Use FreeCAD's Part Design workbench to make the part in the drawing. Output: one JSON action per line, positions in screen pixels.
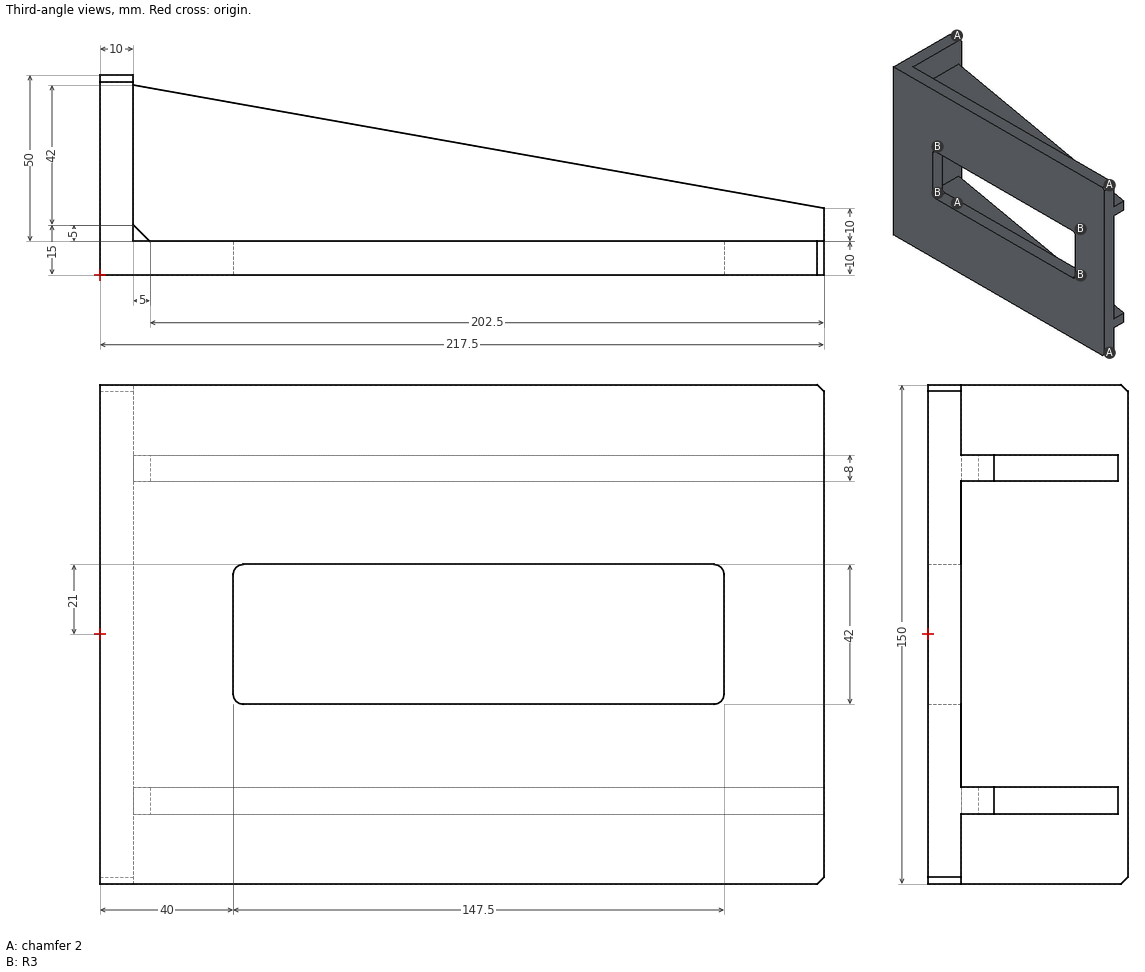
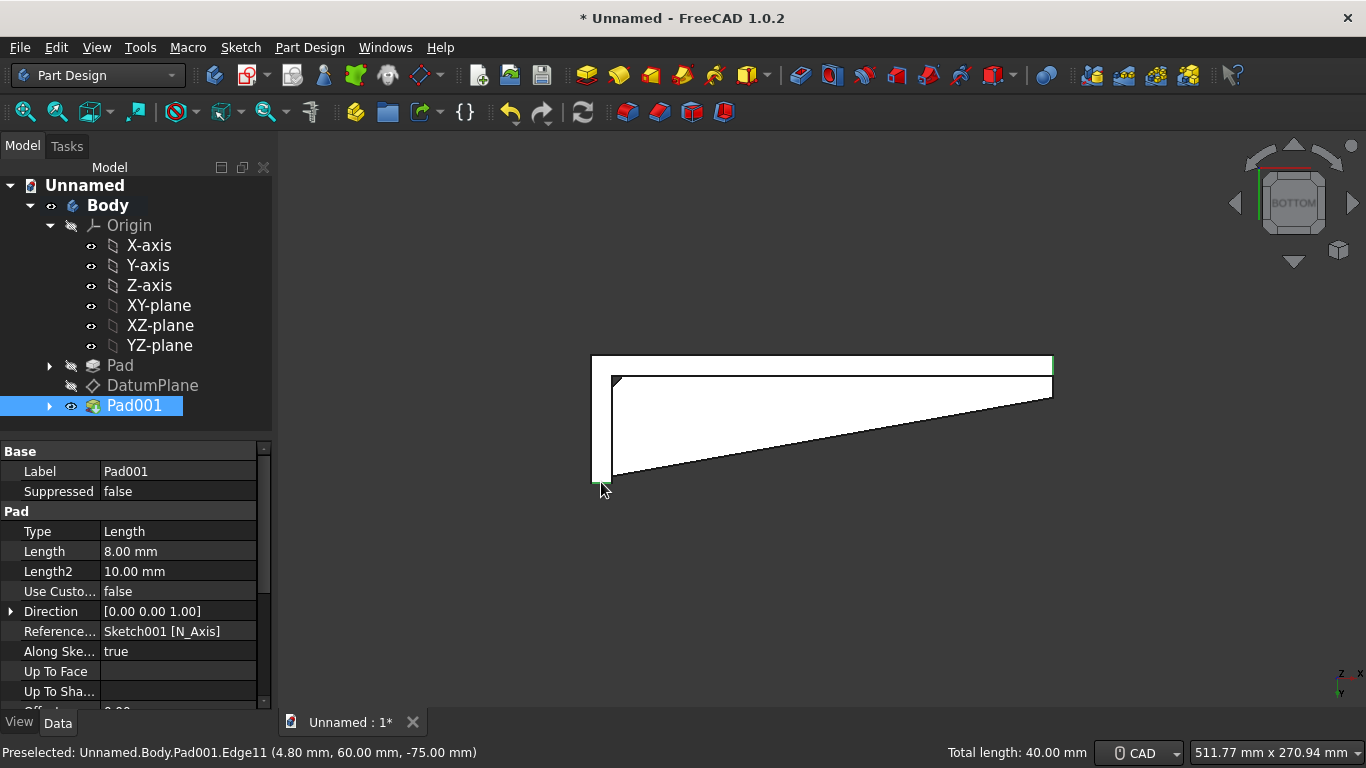
{"action": "left_click", "coordinate": [660, 112]}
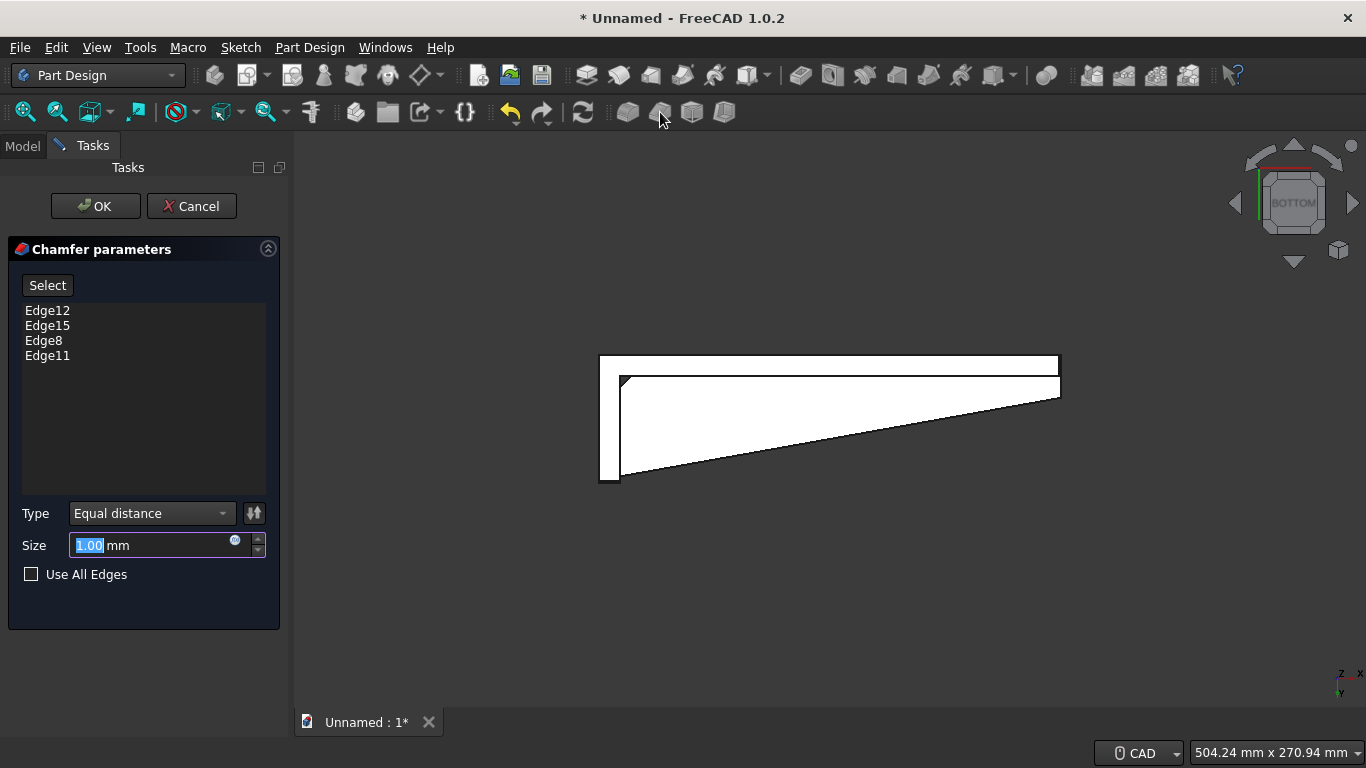
{"action": "type", "text": "2"}
{"action": "key", "text": "Tab"}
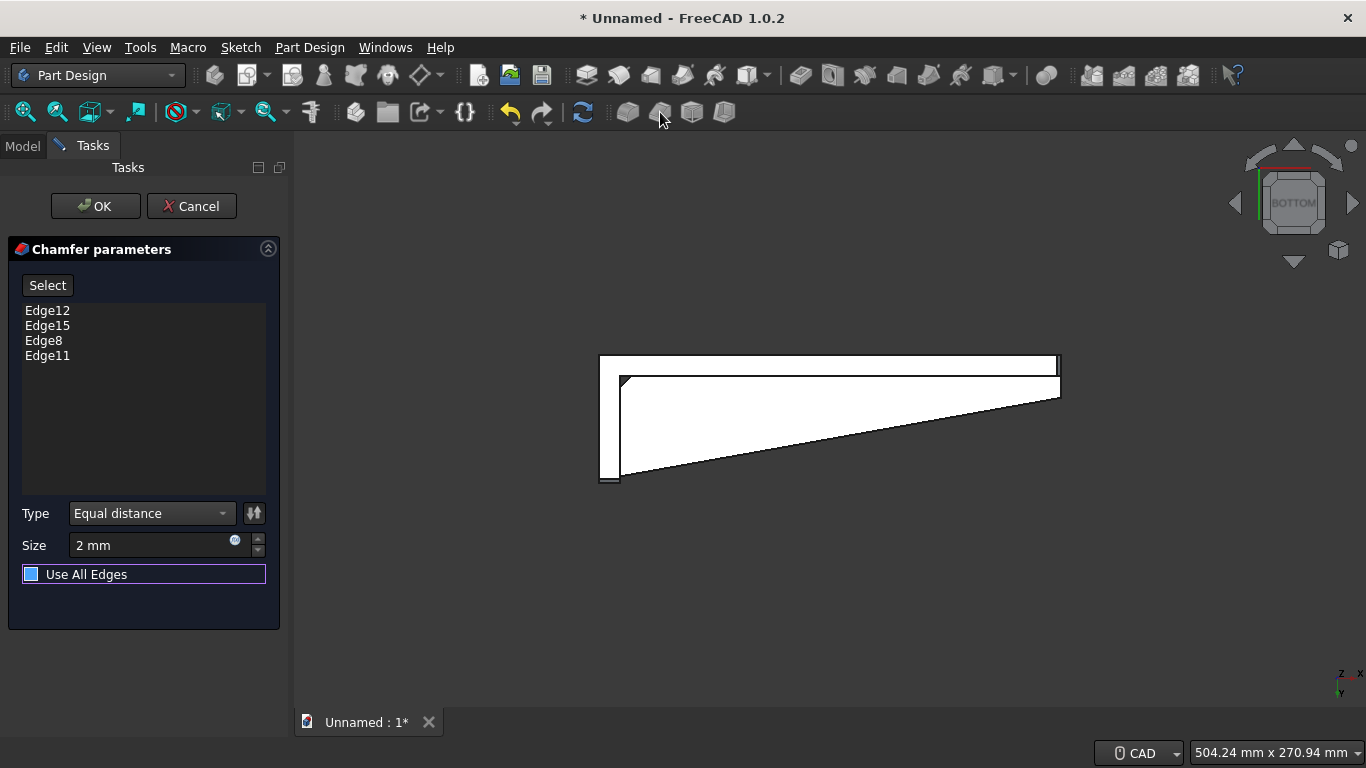
{"action": "left_click", "coordinate": [96, 206]}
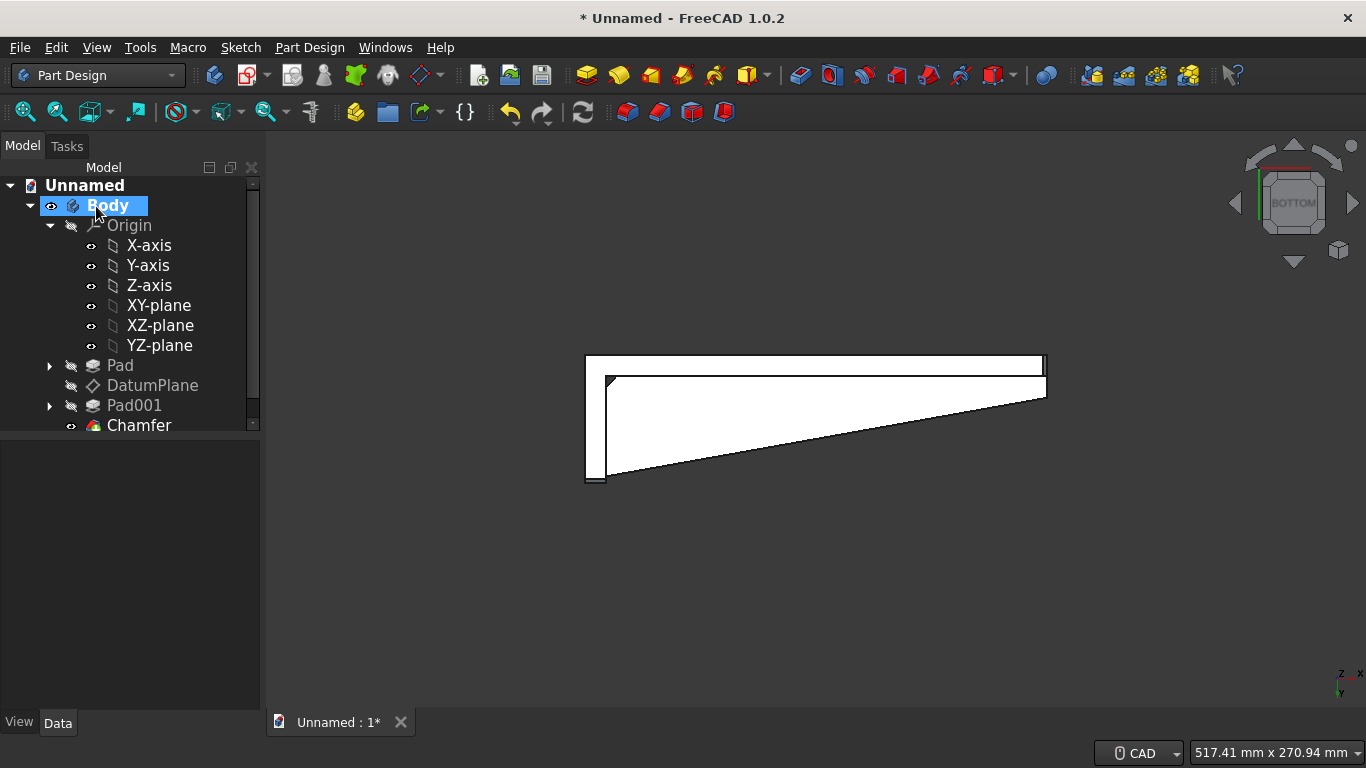
{"action": "left_click", "coordinate": [26, 112]}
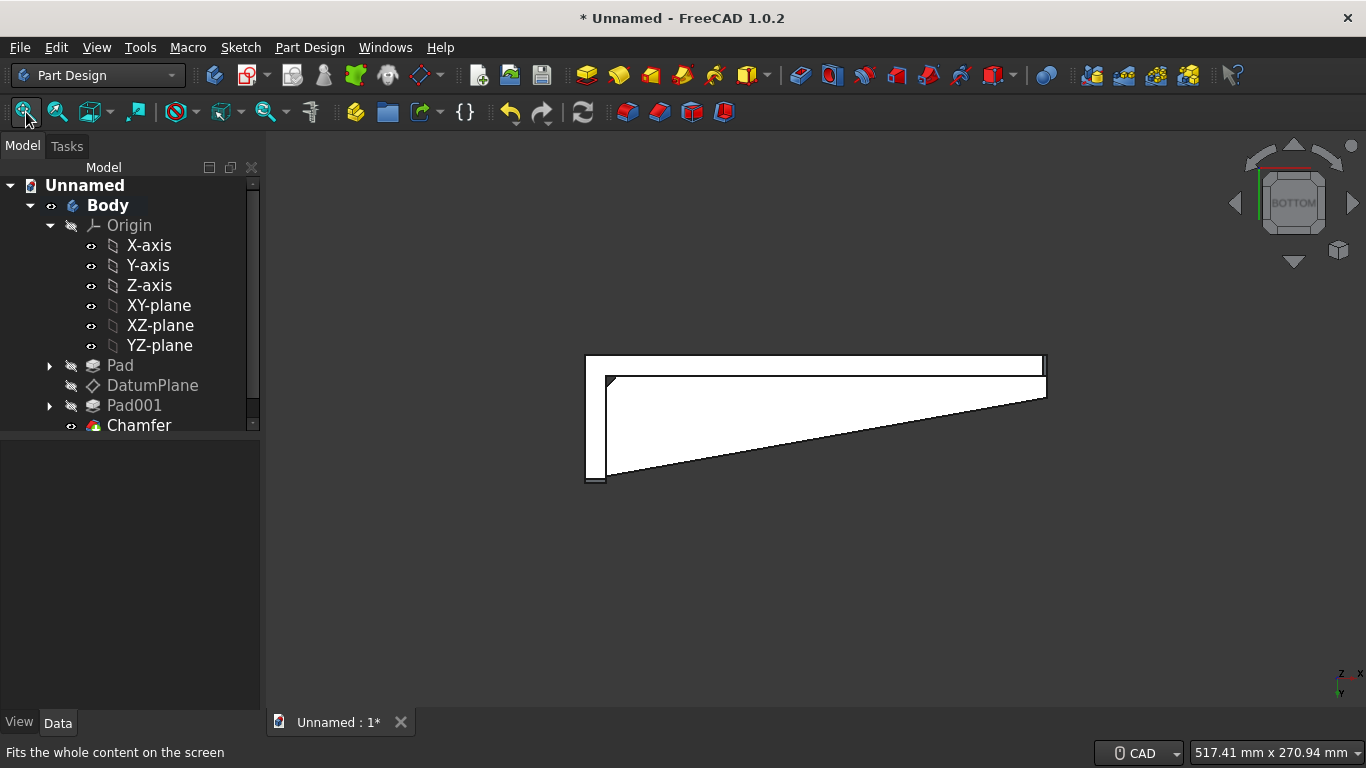
{"action": "left_click", "coordinate": [116, 406]}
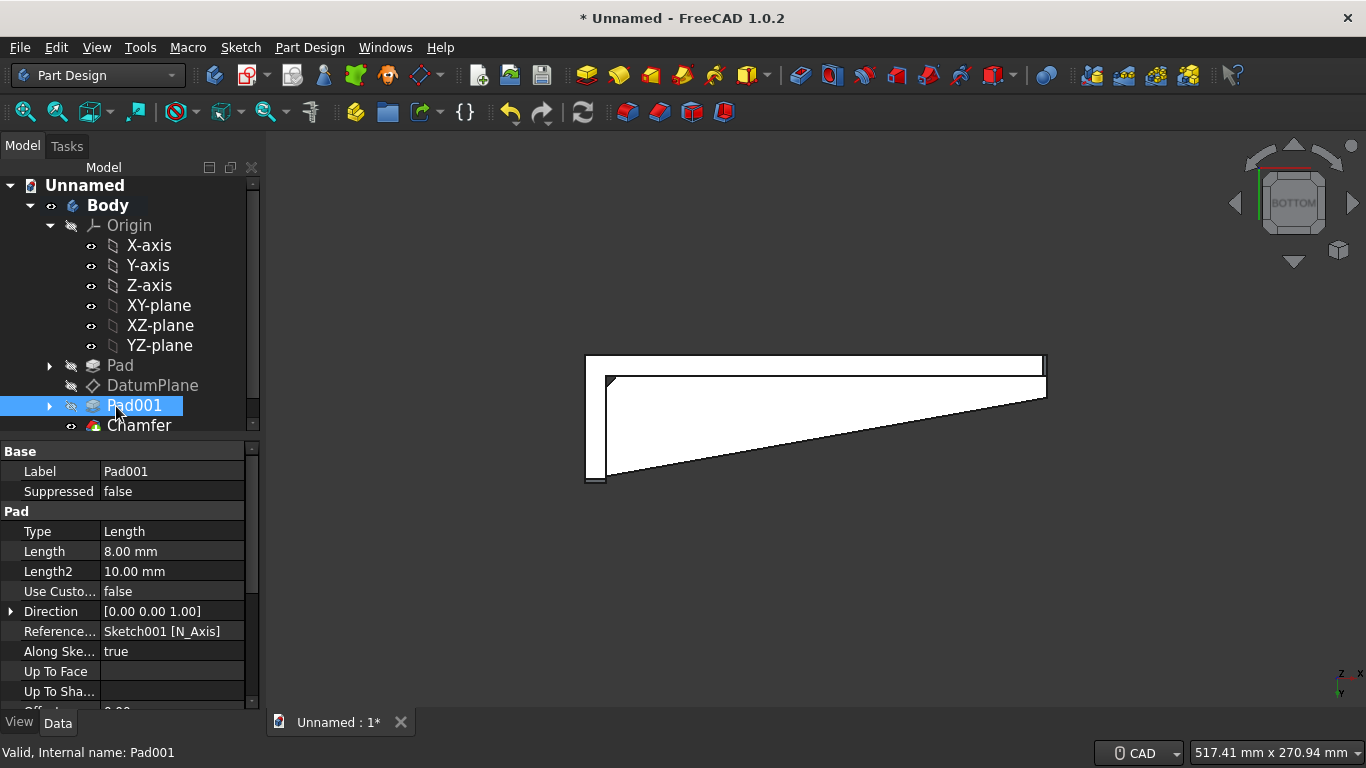
{"action": "left_click", "coordinate": [1092, 76]}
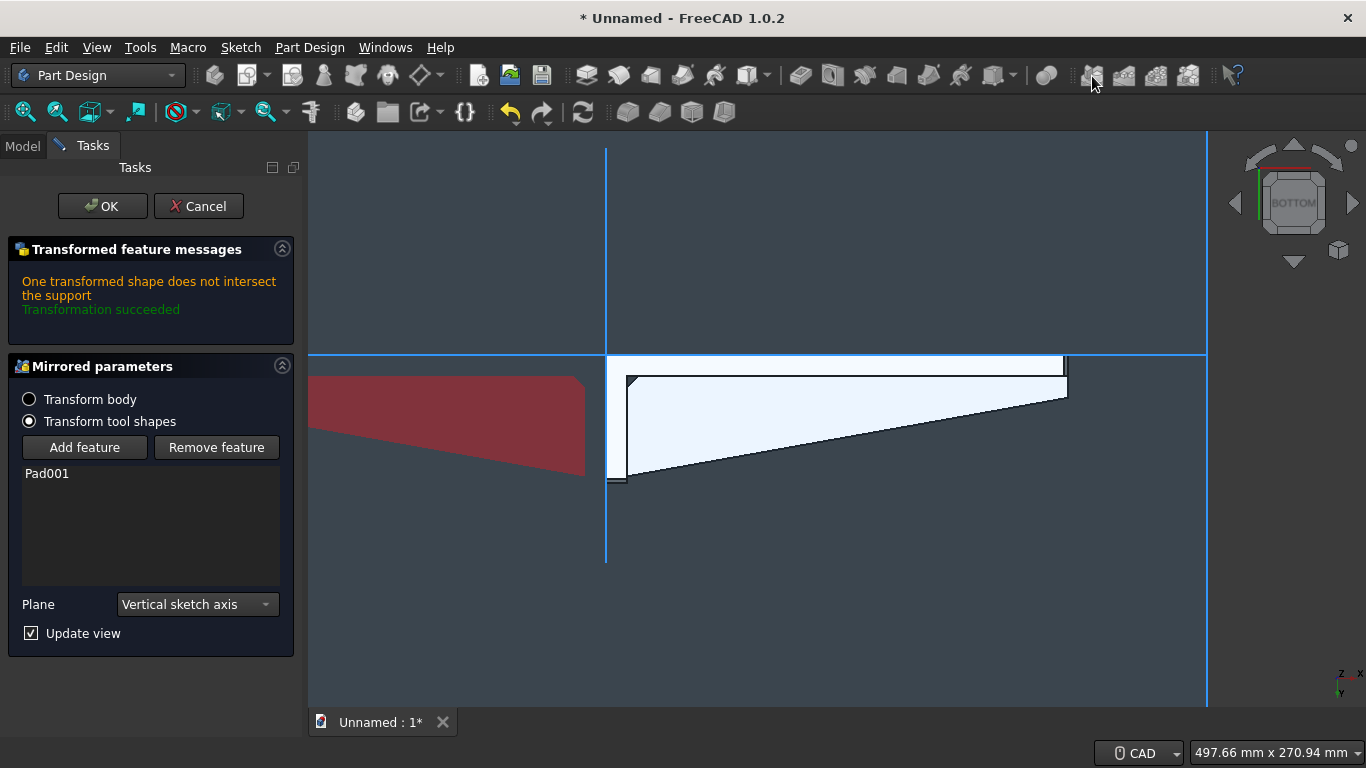
{"action": "left_click", "coordinate": [198, 604]}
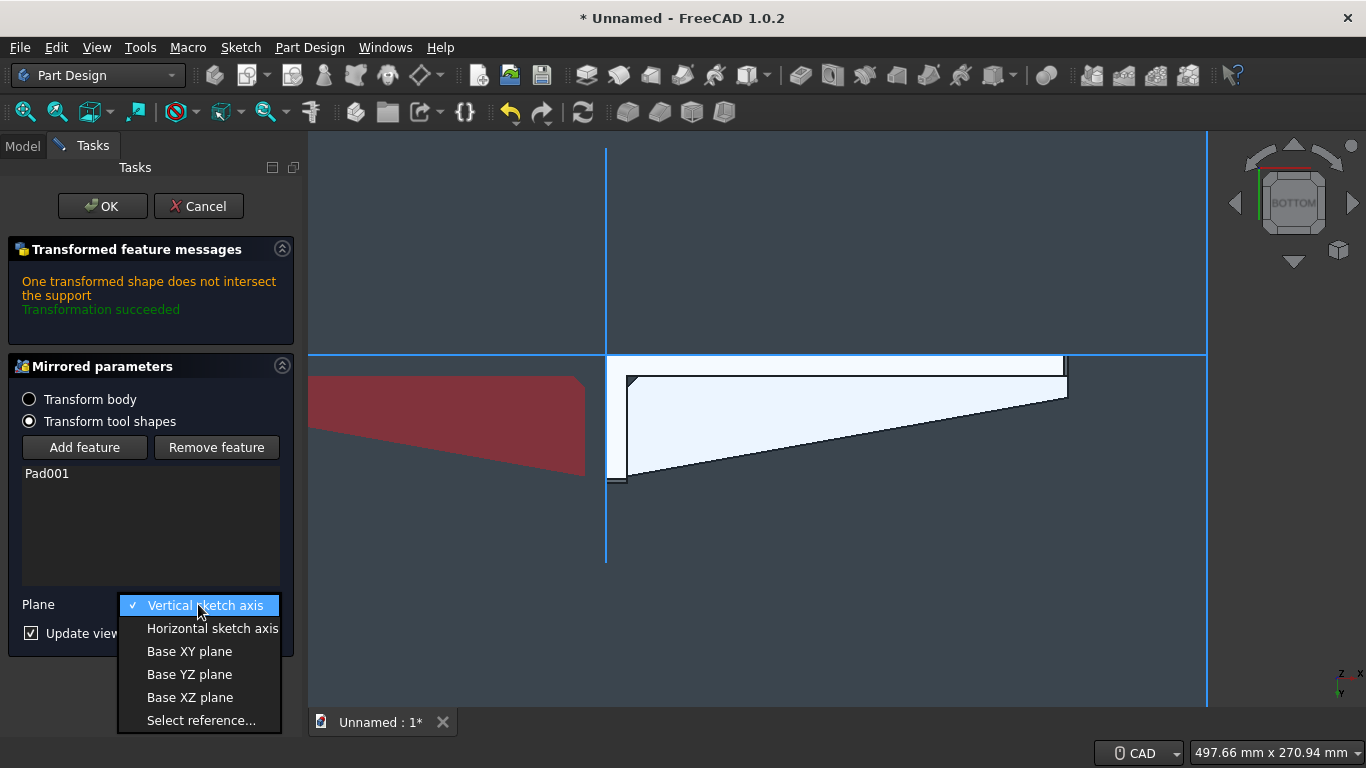
{"action": "left_click", "coordinate": [198, 652]}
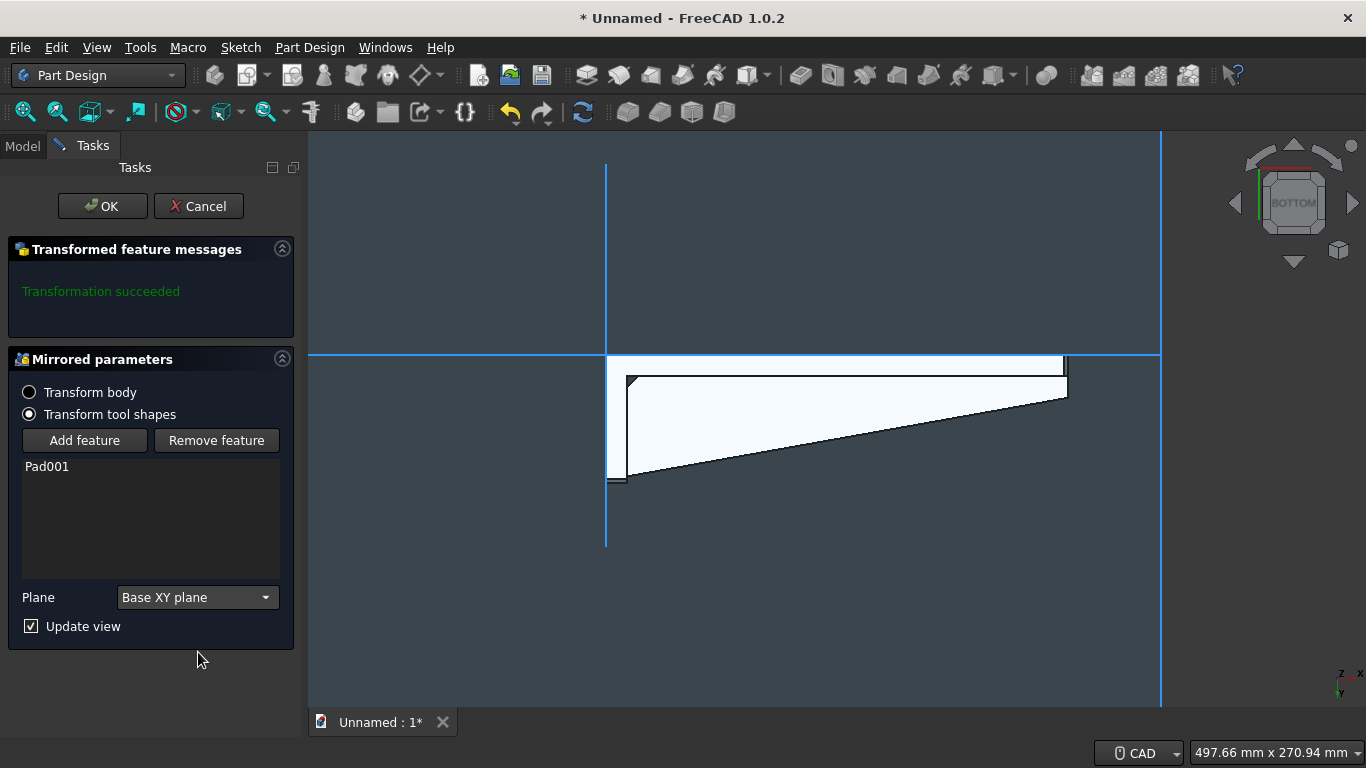
{"action": "left_click", "coordinate": [103, 206]}